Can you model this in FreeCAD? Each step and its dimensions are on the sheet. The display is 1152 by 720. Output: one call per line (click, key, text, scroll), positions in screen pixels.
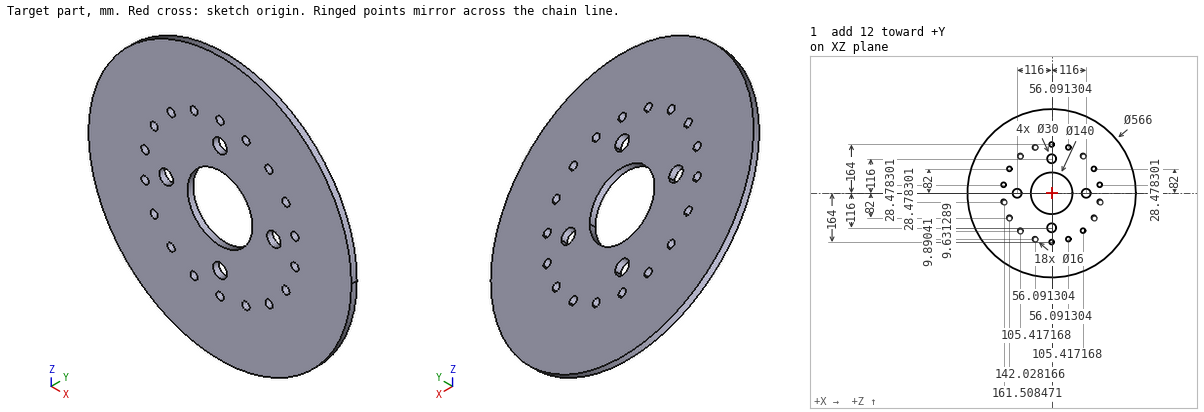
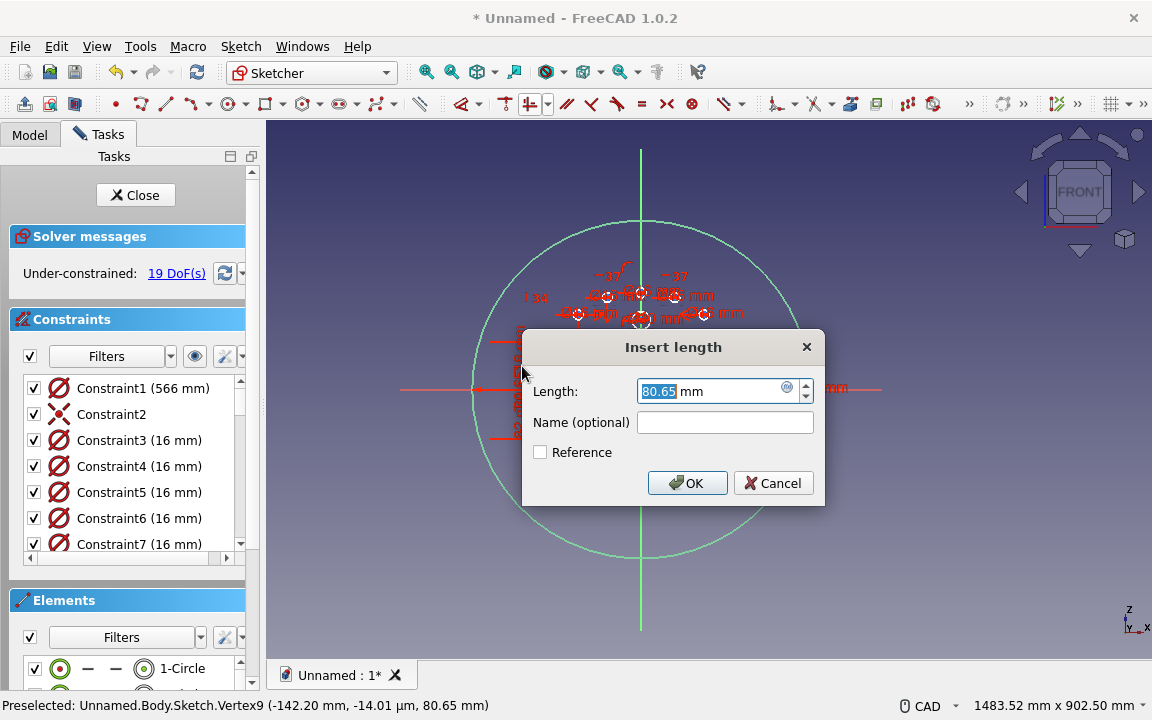
text(82)
key(Return)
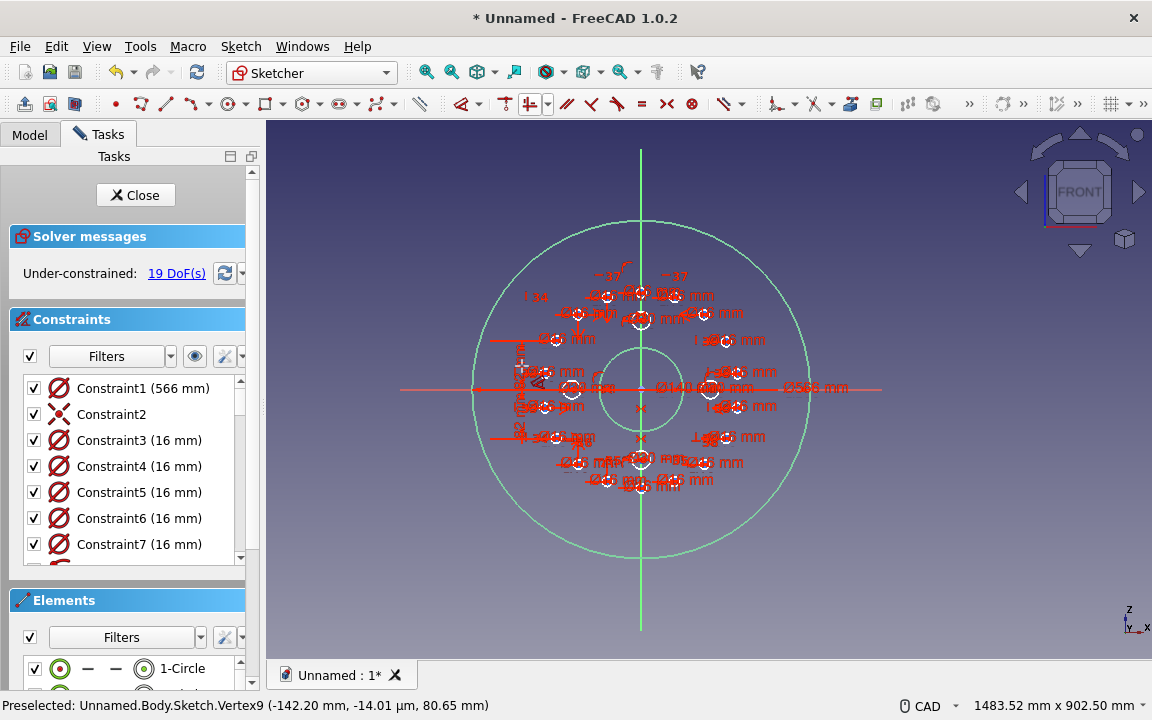
click(726, 342)
click(760, 366)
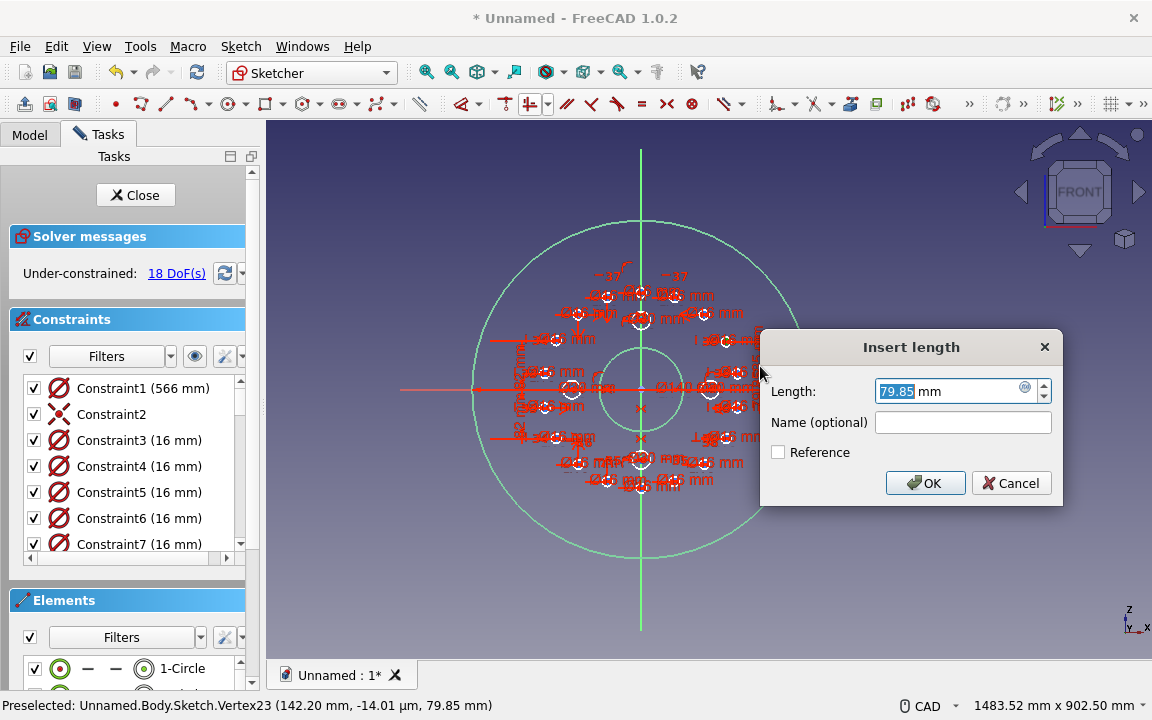
text(82)
key(Return)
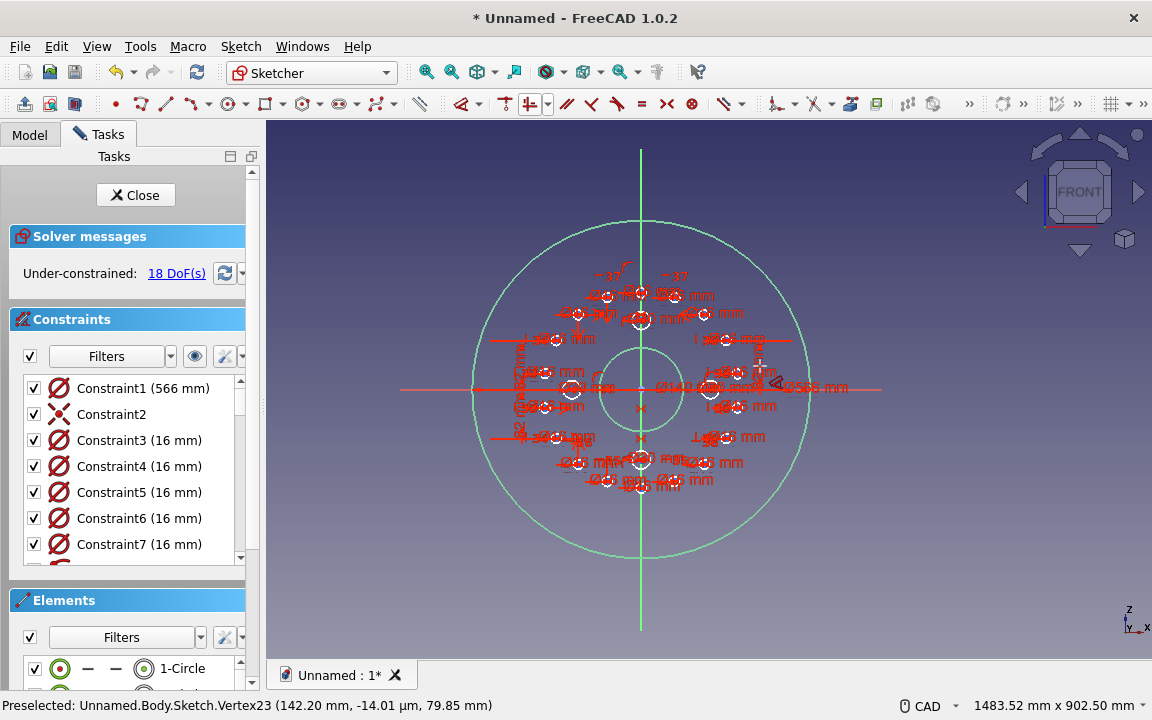
click(641, 488)
click(675, 439)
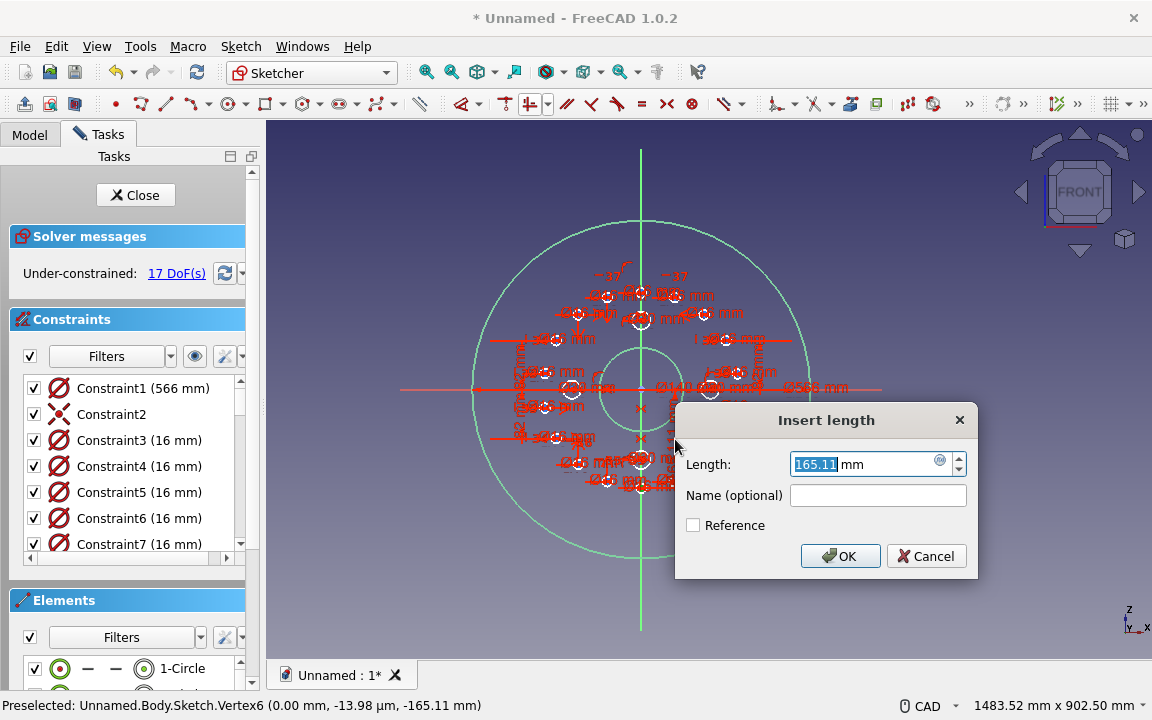
text(164)
key(Return)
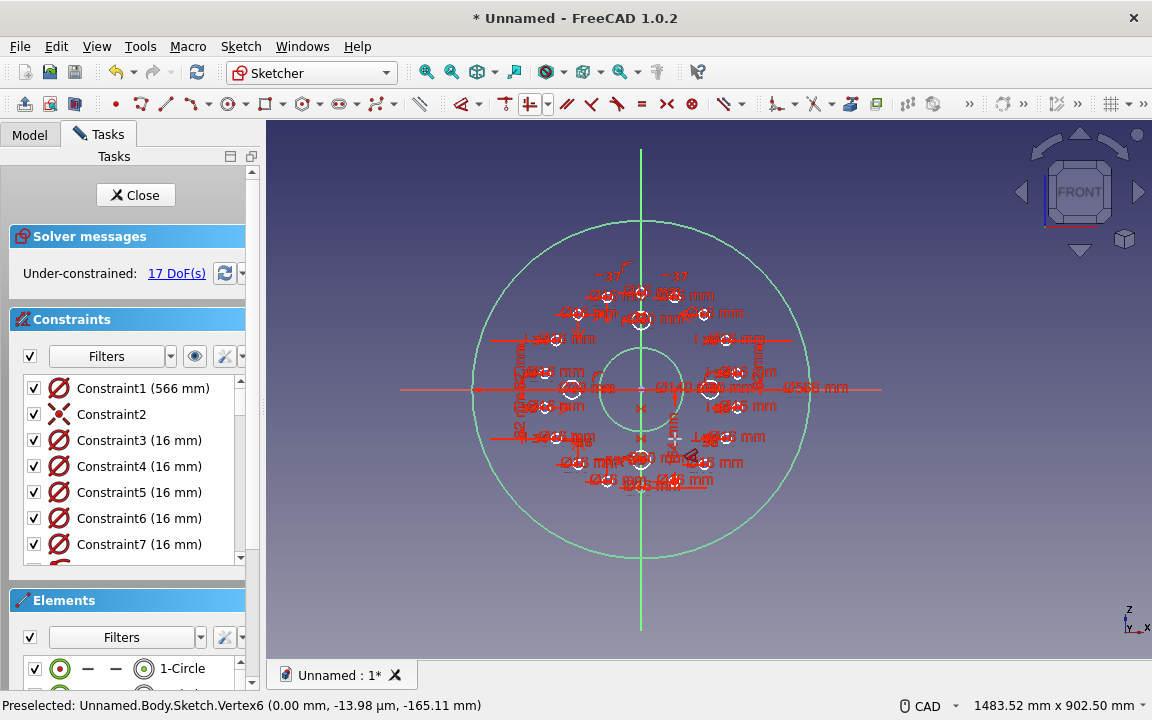
click(641, 460)
click(699, 409)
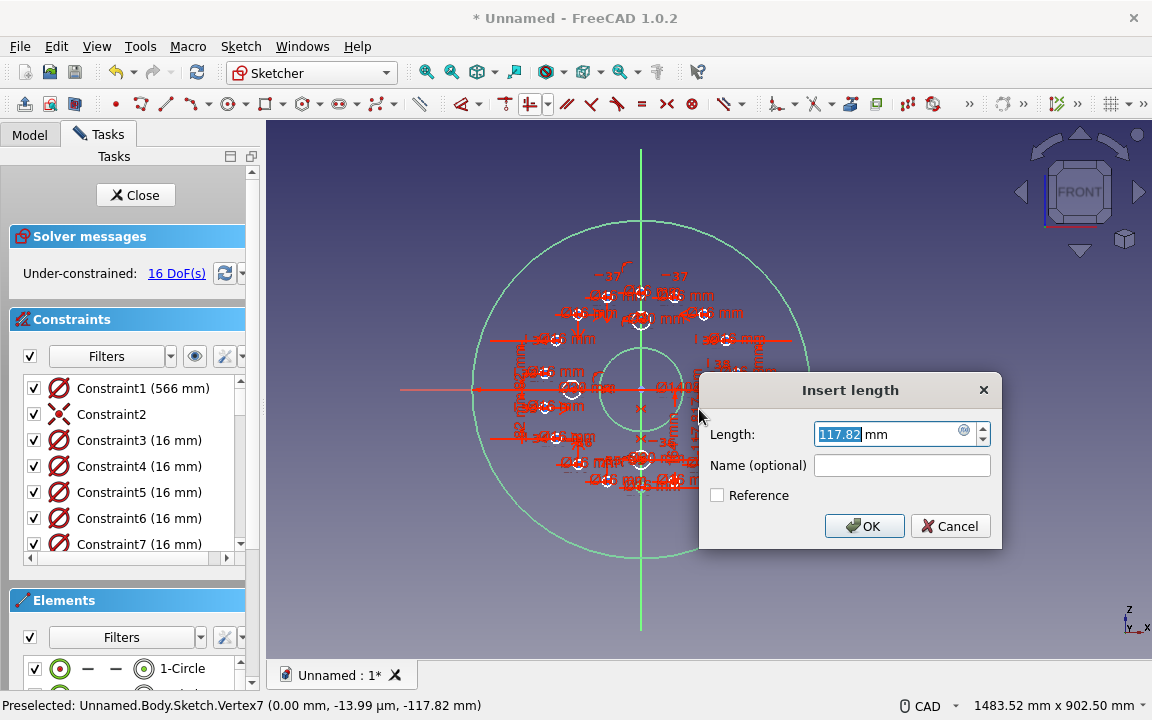
text(116)
key(Return)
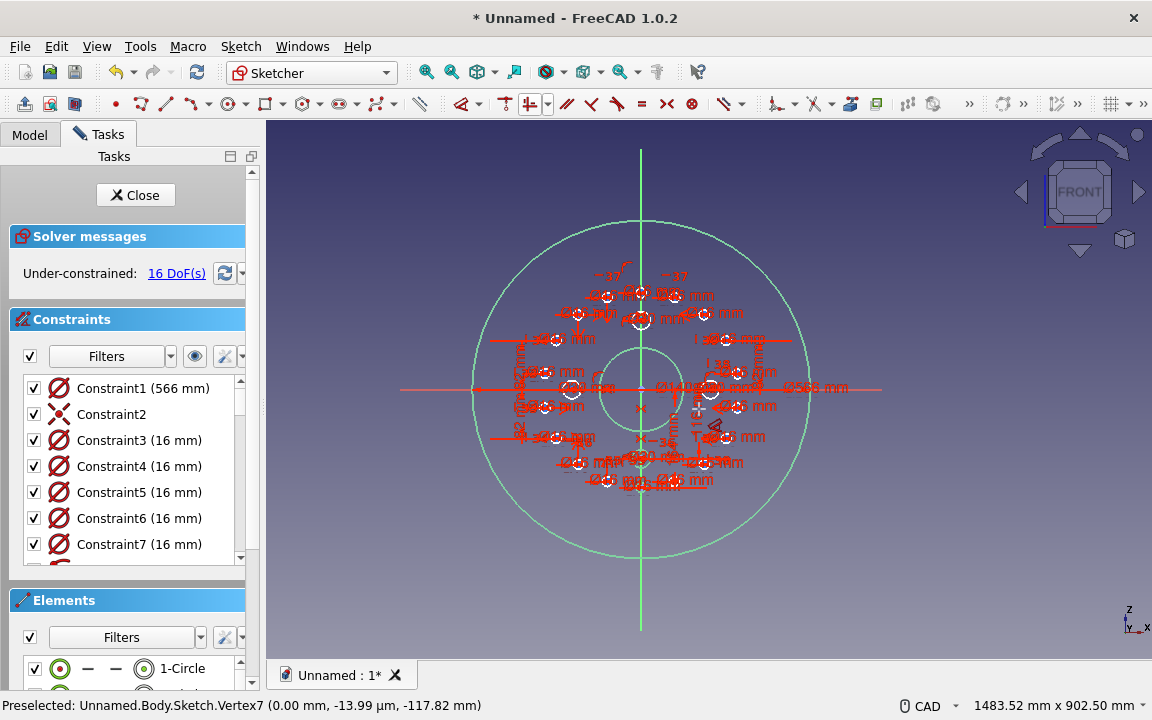
click(572, 390)
click(591, 448)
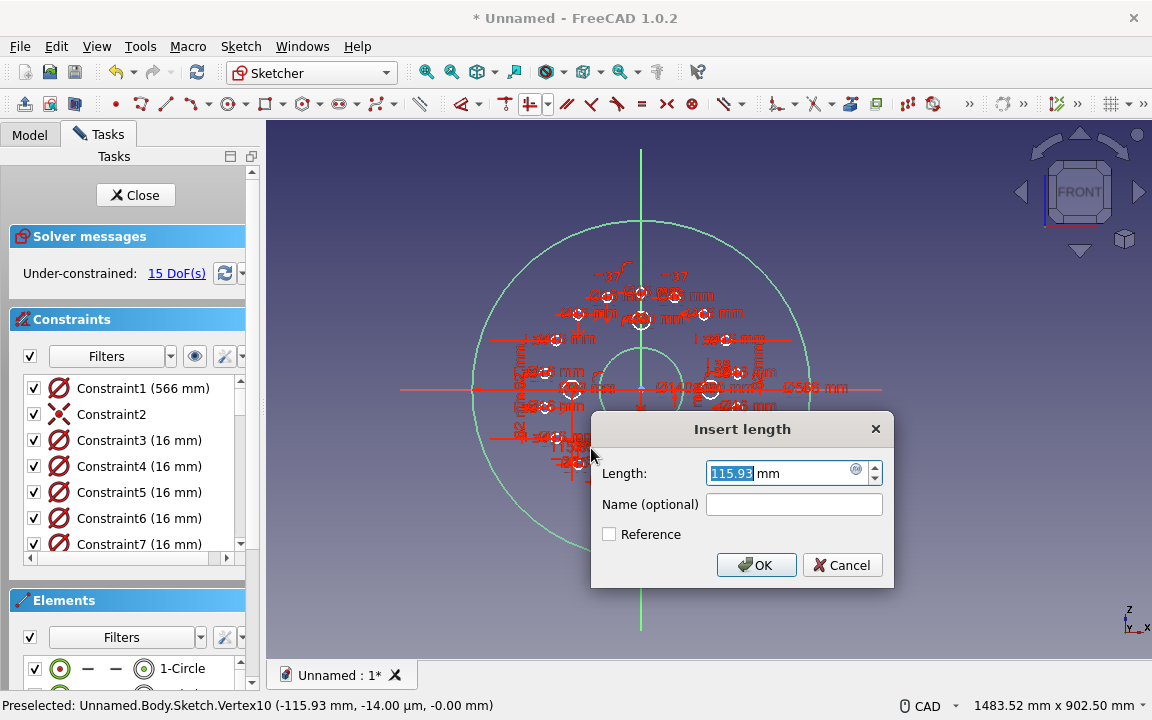
text(116)
key(Return)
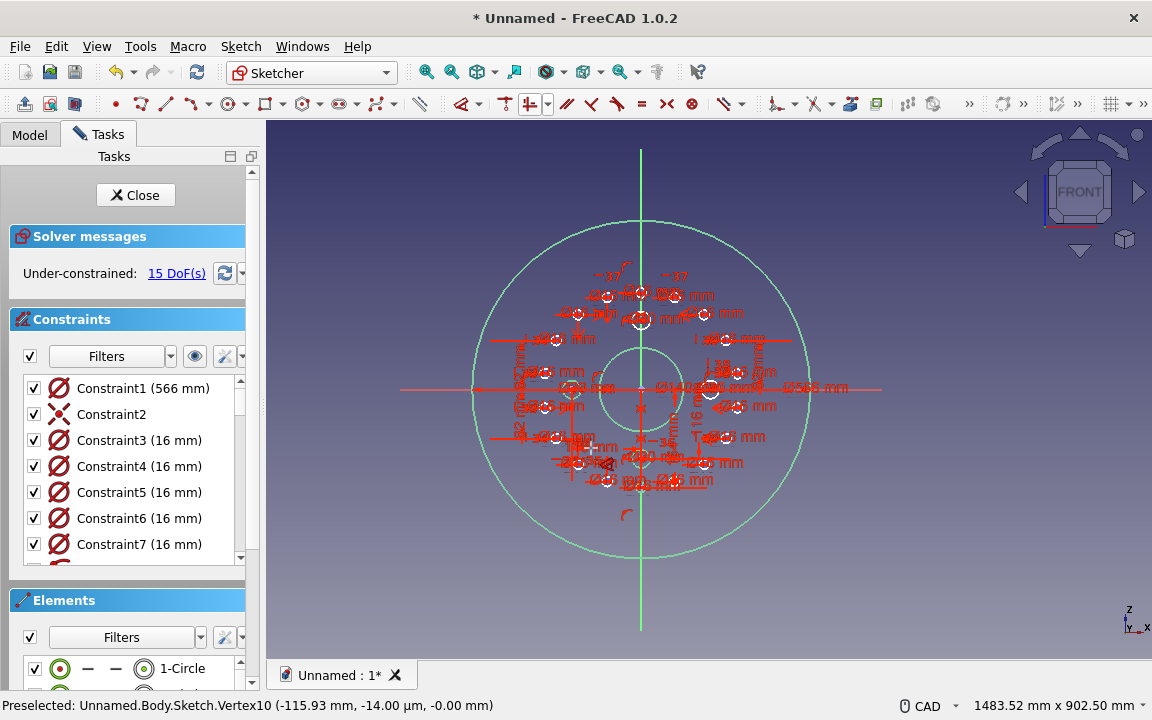
click(710, 390)
click(676, 332)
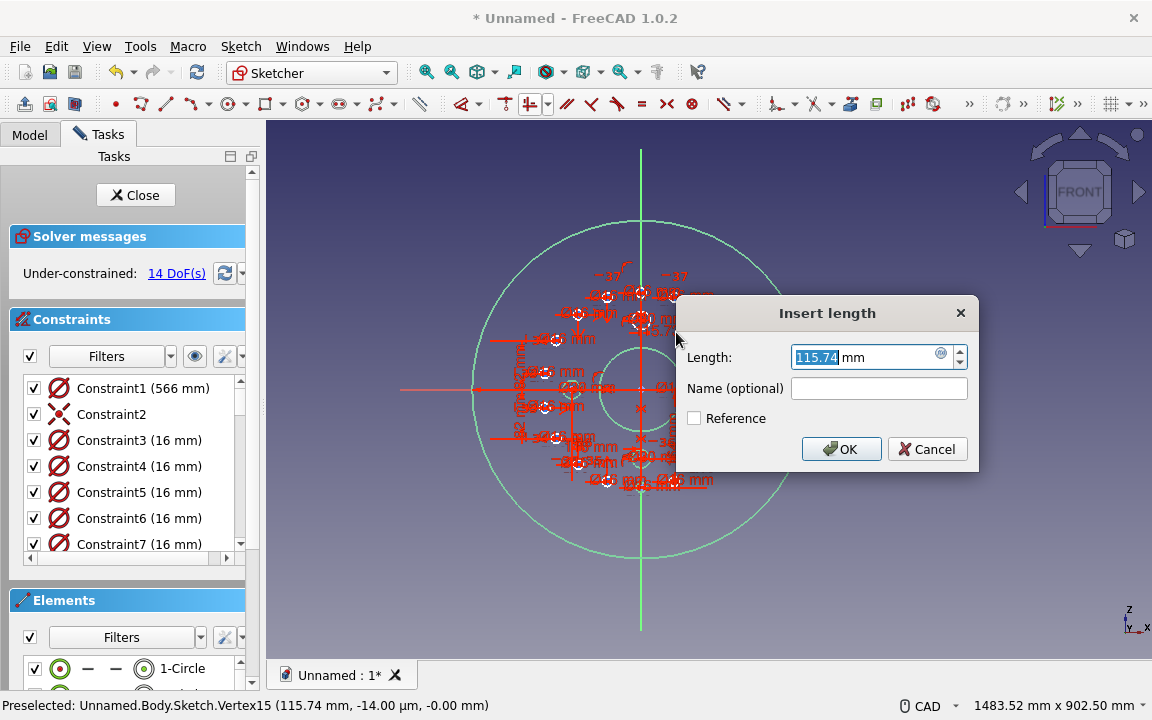
text(116)
key(Return)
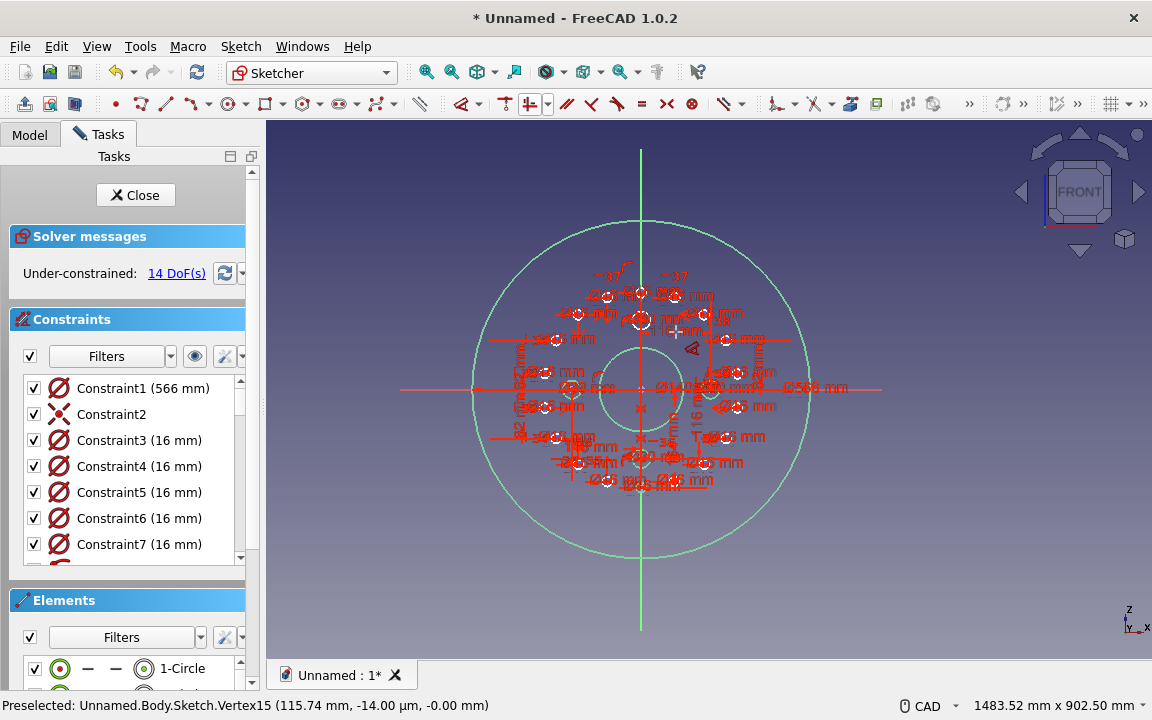
click(641, 321)
click(583, 339)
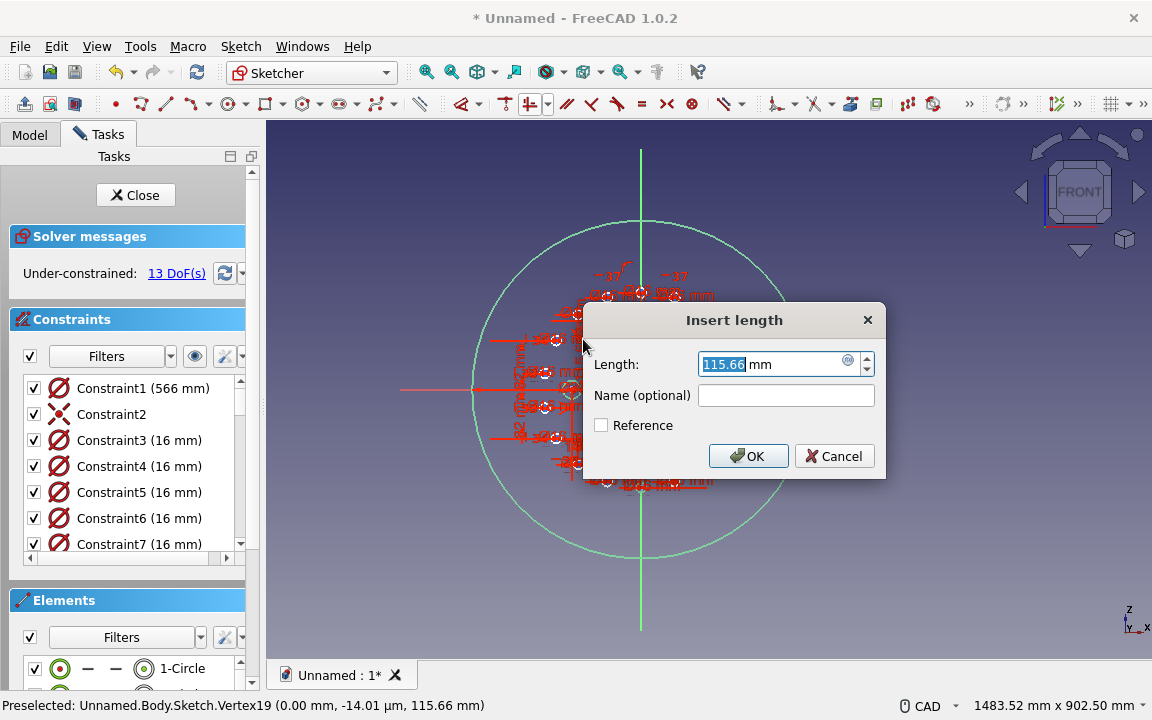
text(116)
key(Return)